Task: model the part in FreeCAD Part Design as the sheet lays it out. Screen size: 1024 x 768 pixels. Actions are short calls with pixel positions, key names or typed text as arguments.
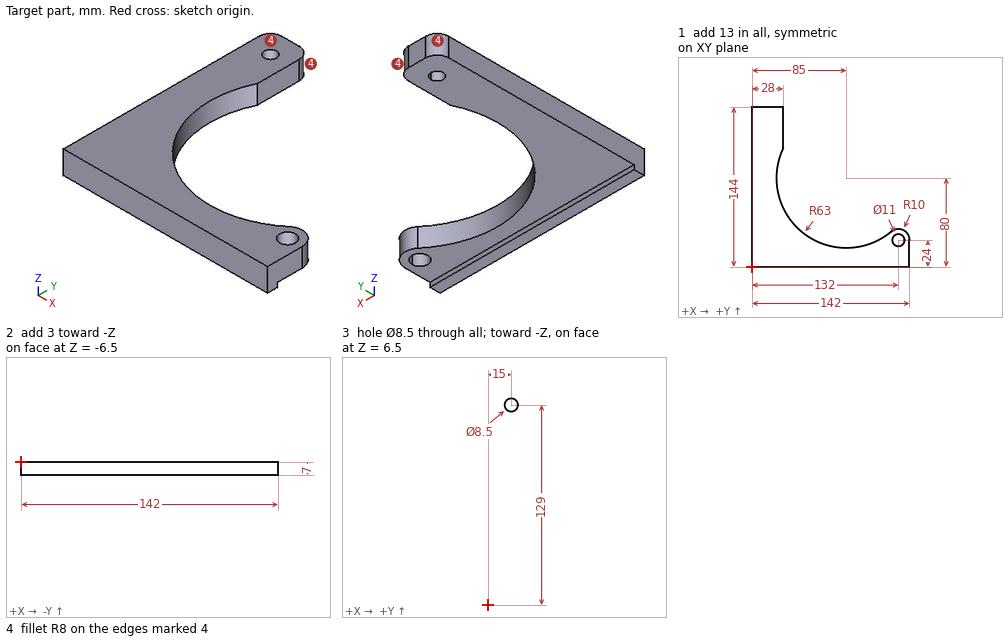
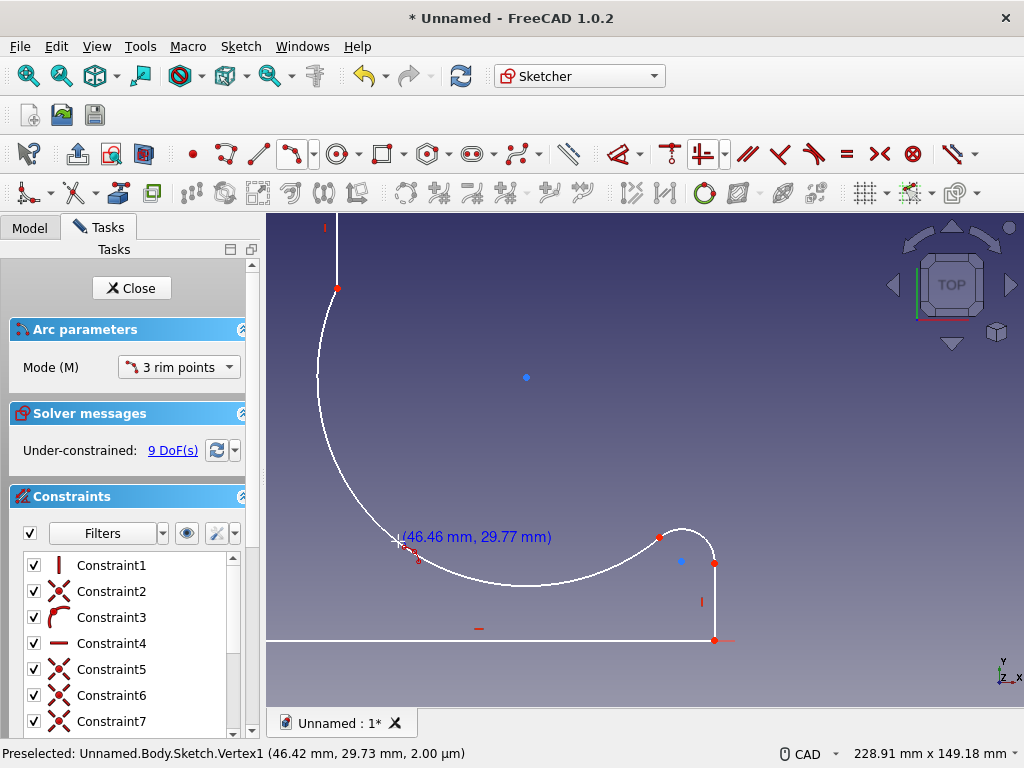
click(336, 154)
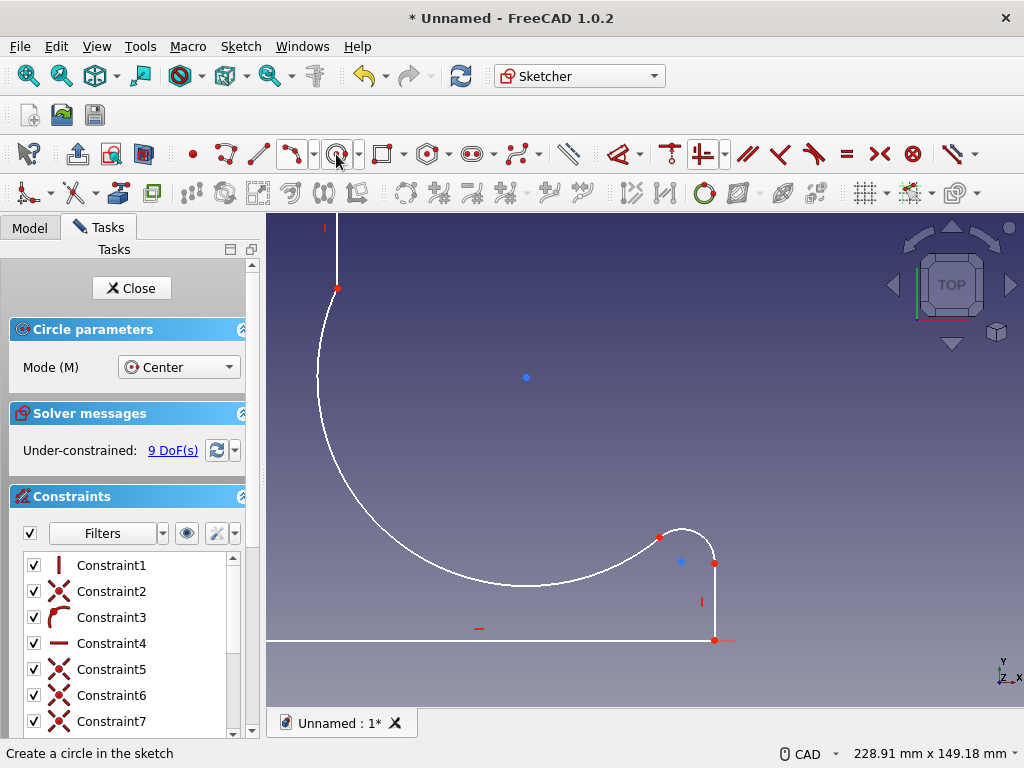
scroll(681, 561, up, 18)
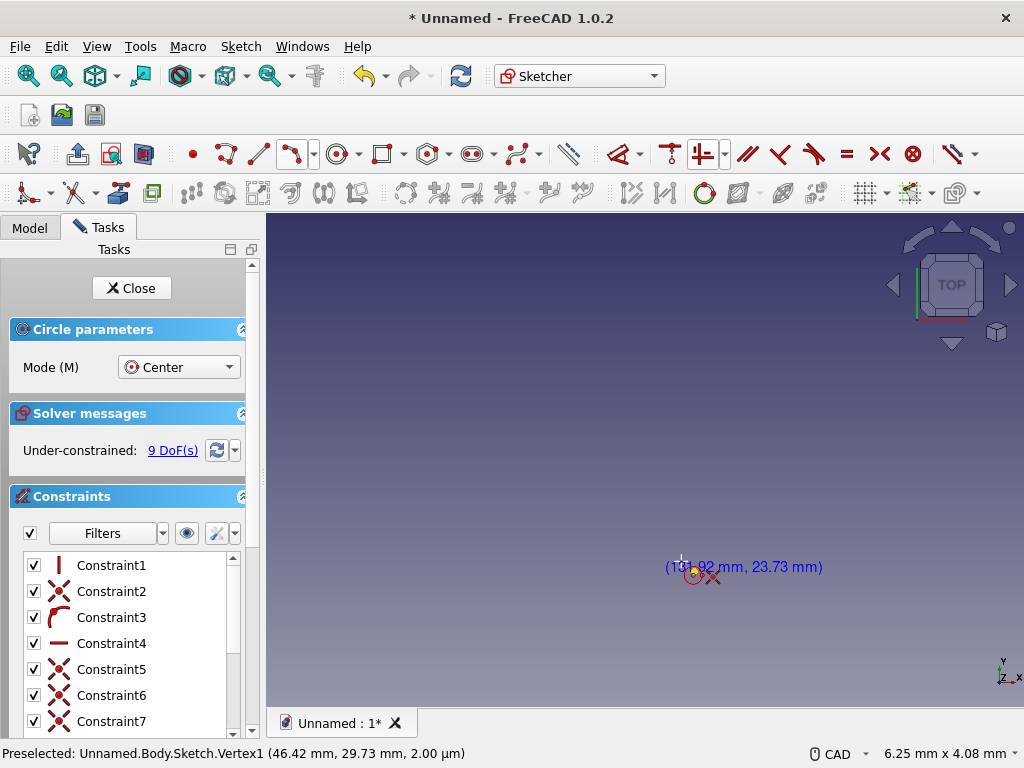
click(671, 540)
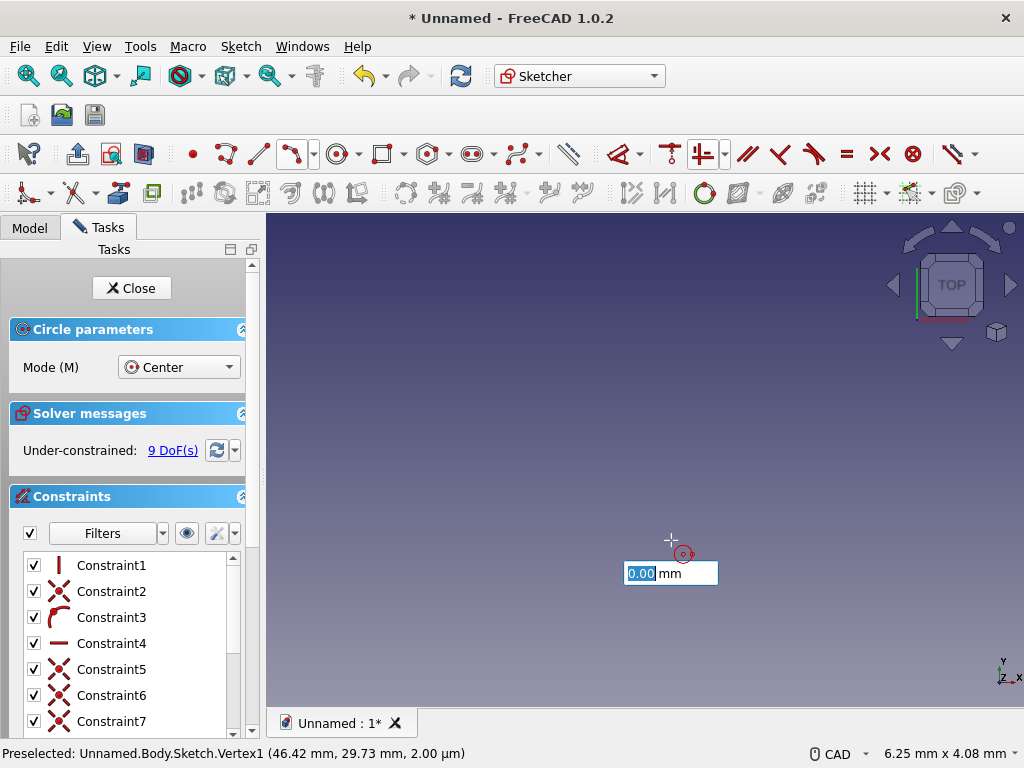
scroll(576, 460, down, 15)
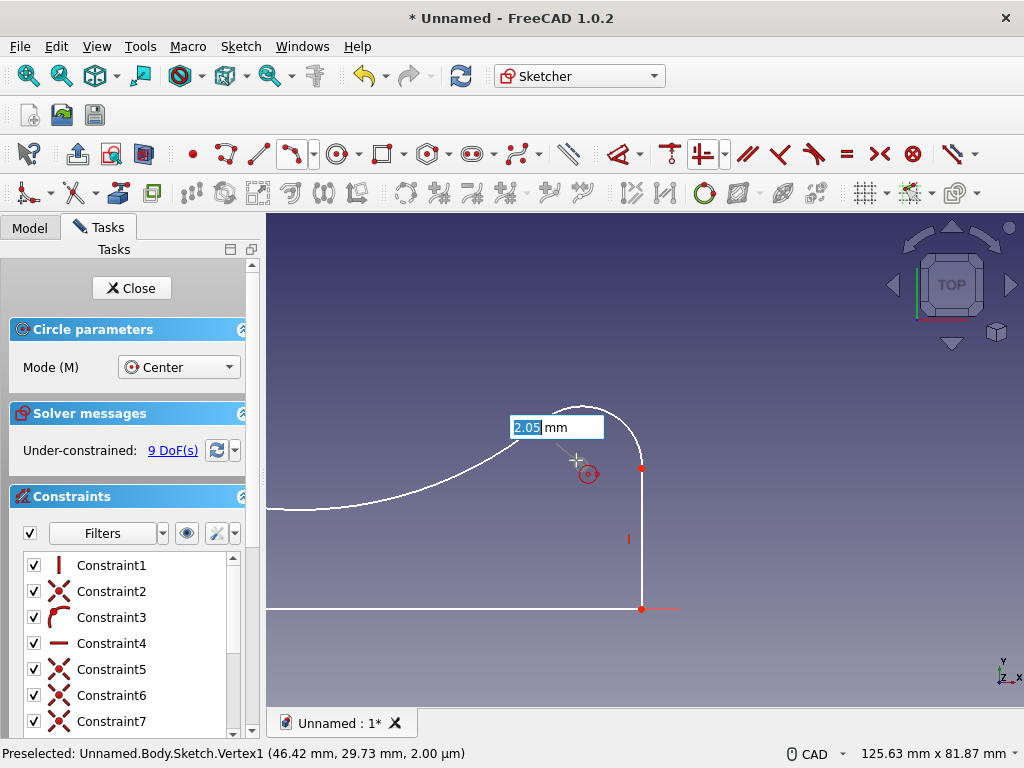
scroll(788, 626, down, 5)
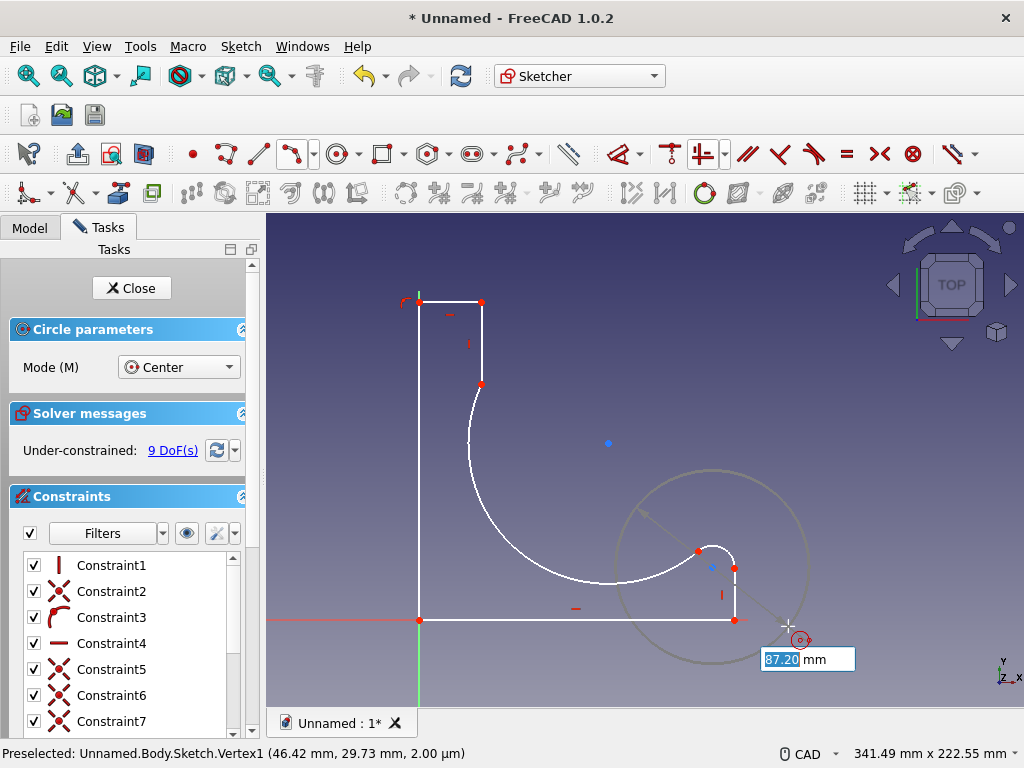
scroll(721, 558, up, 3)
move(720, 558)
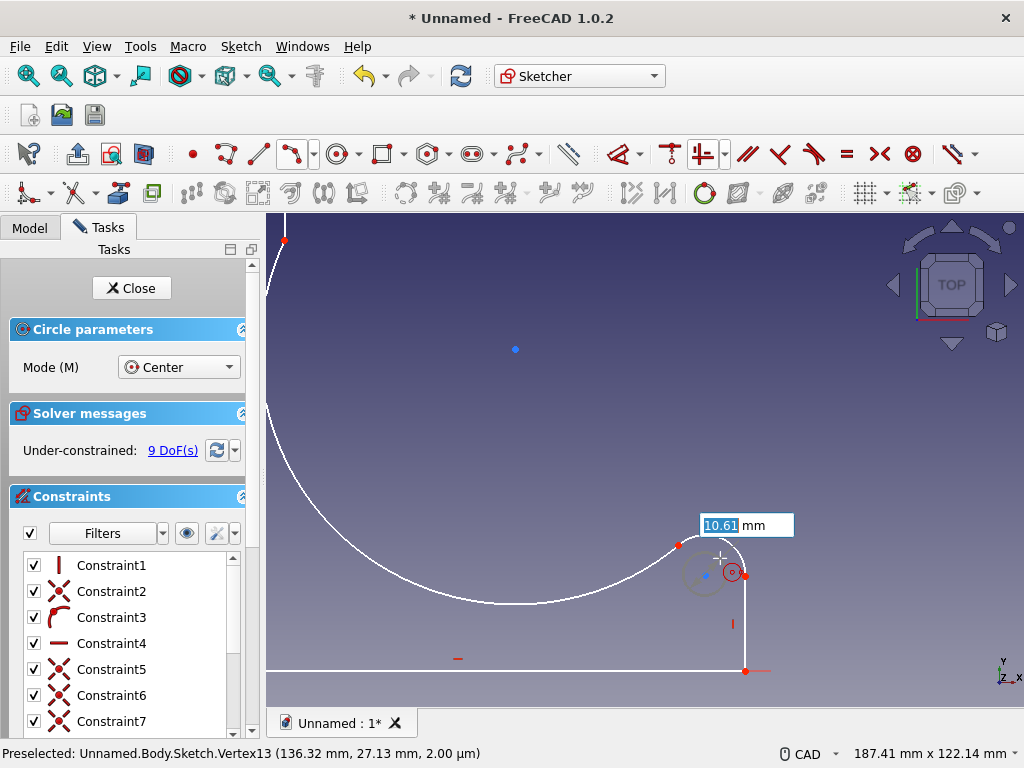
text(11)
key(Return)
key(Escape)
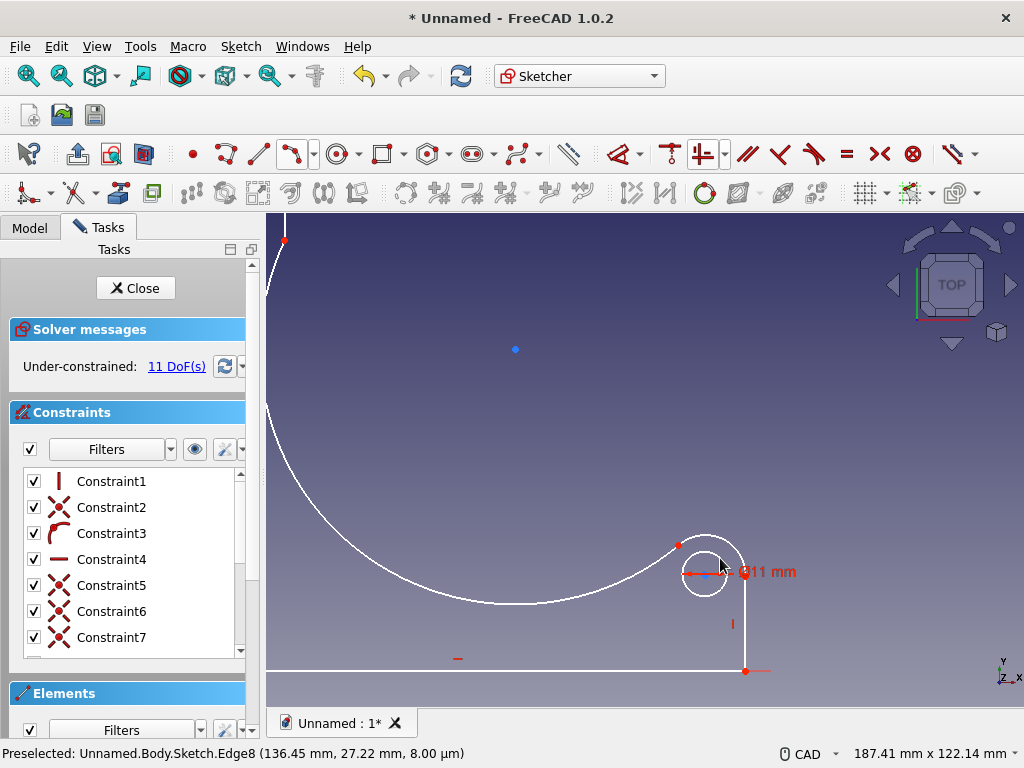
click(745, 643)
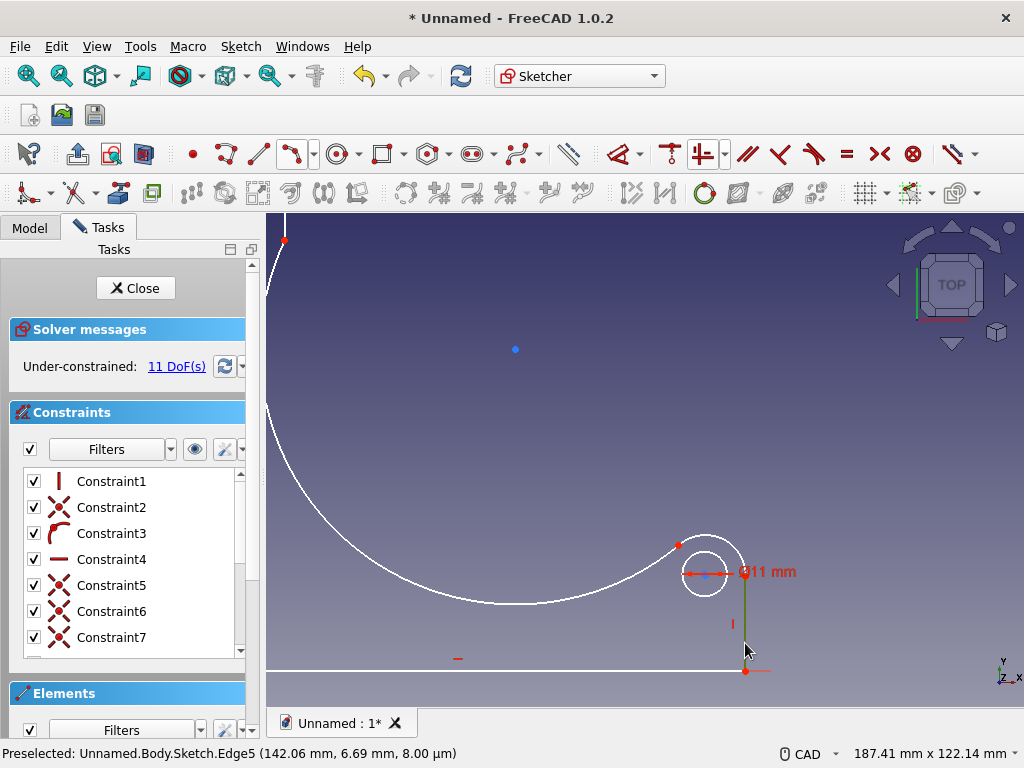
click(737, 550)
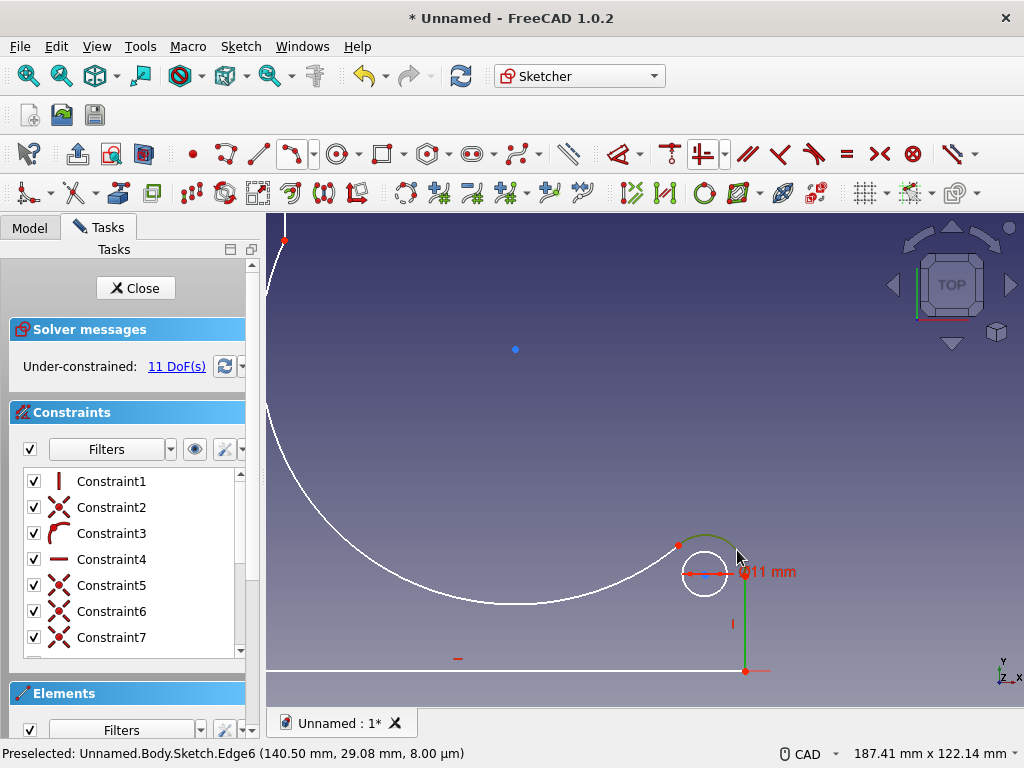
click(814, 154)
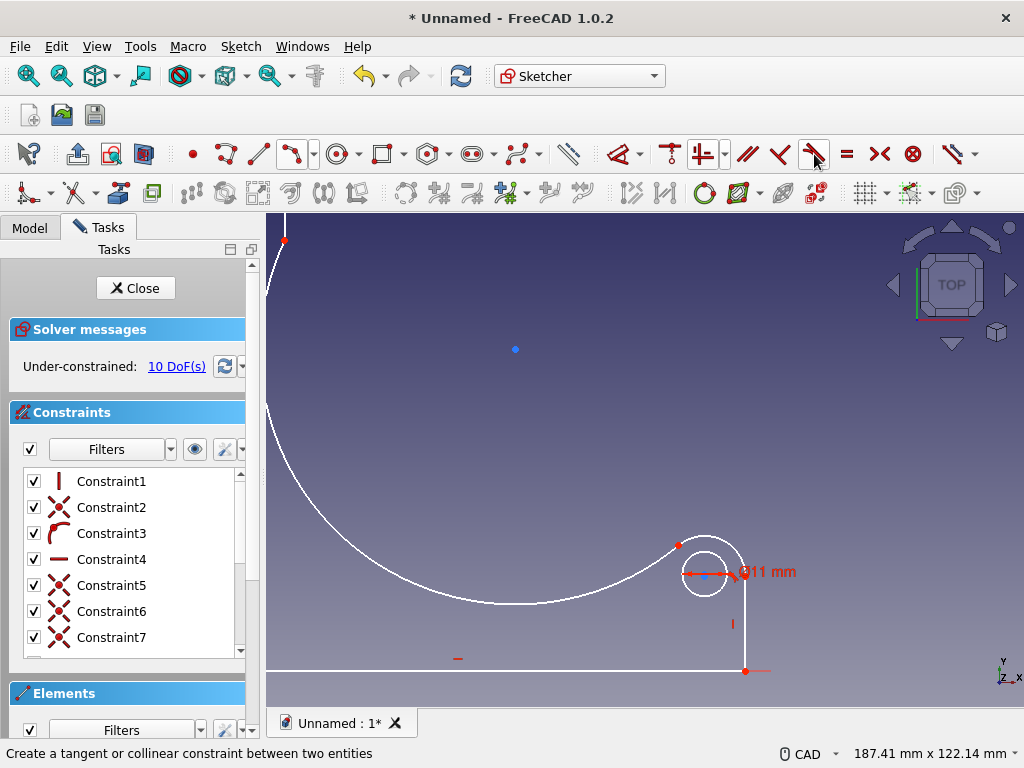
click(736, 551)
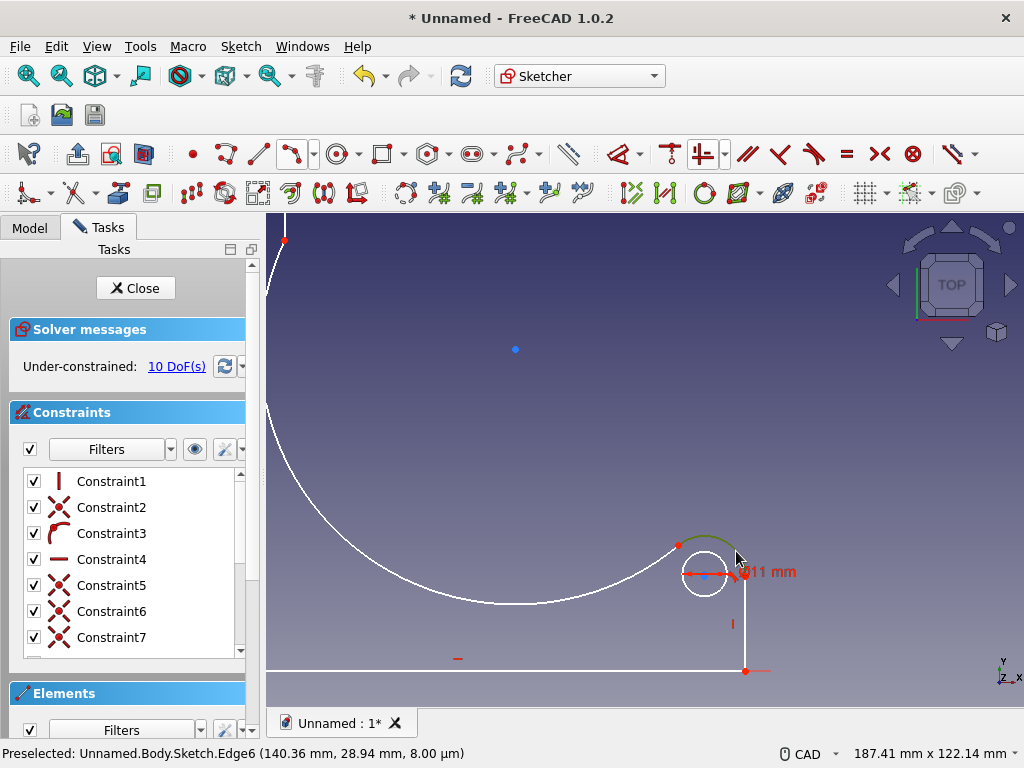
click(486, 603)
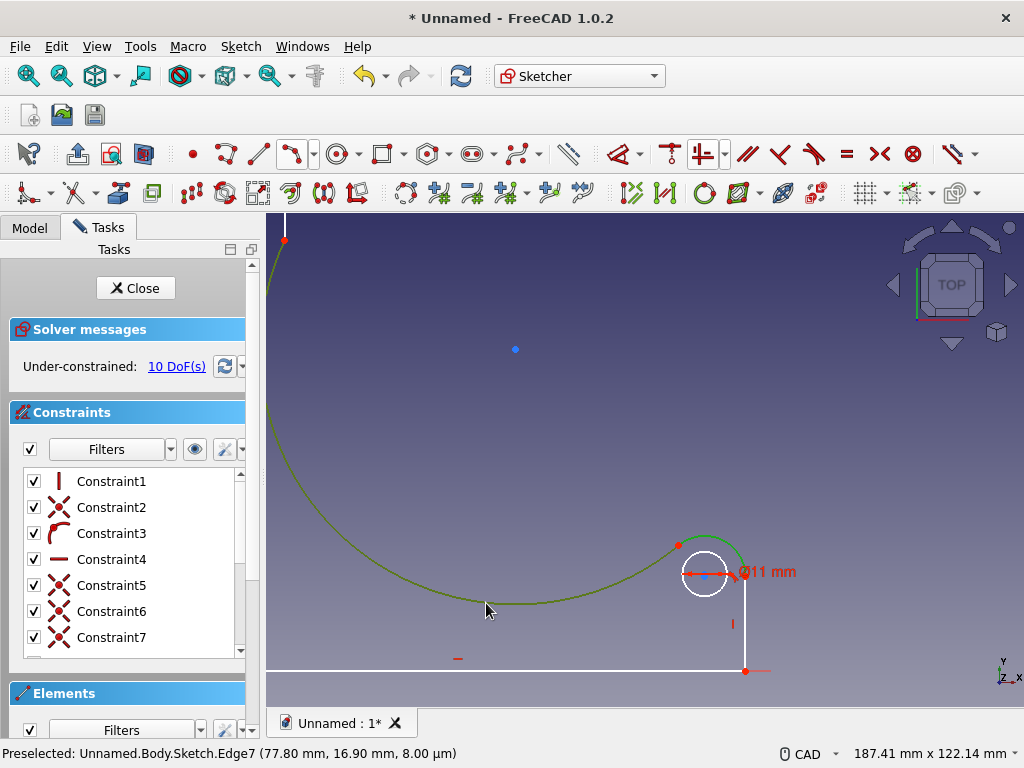
click(814, 154)